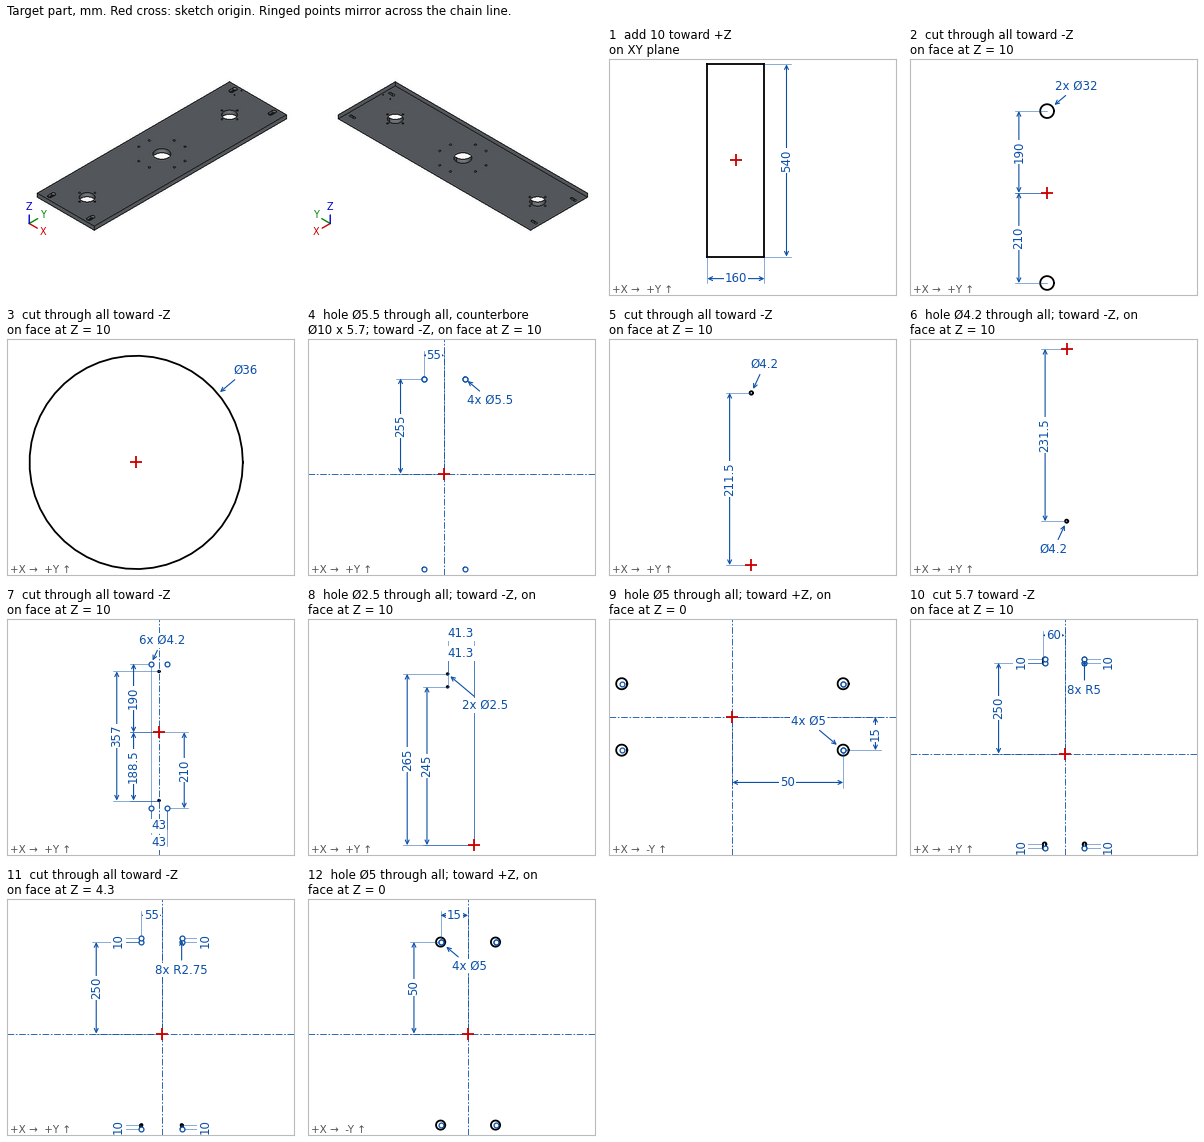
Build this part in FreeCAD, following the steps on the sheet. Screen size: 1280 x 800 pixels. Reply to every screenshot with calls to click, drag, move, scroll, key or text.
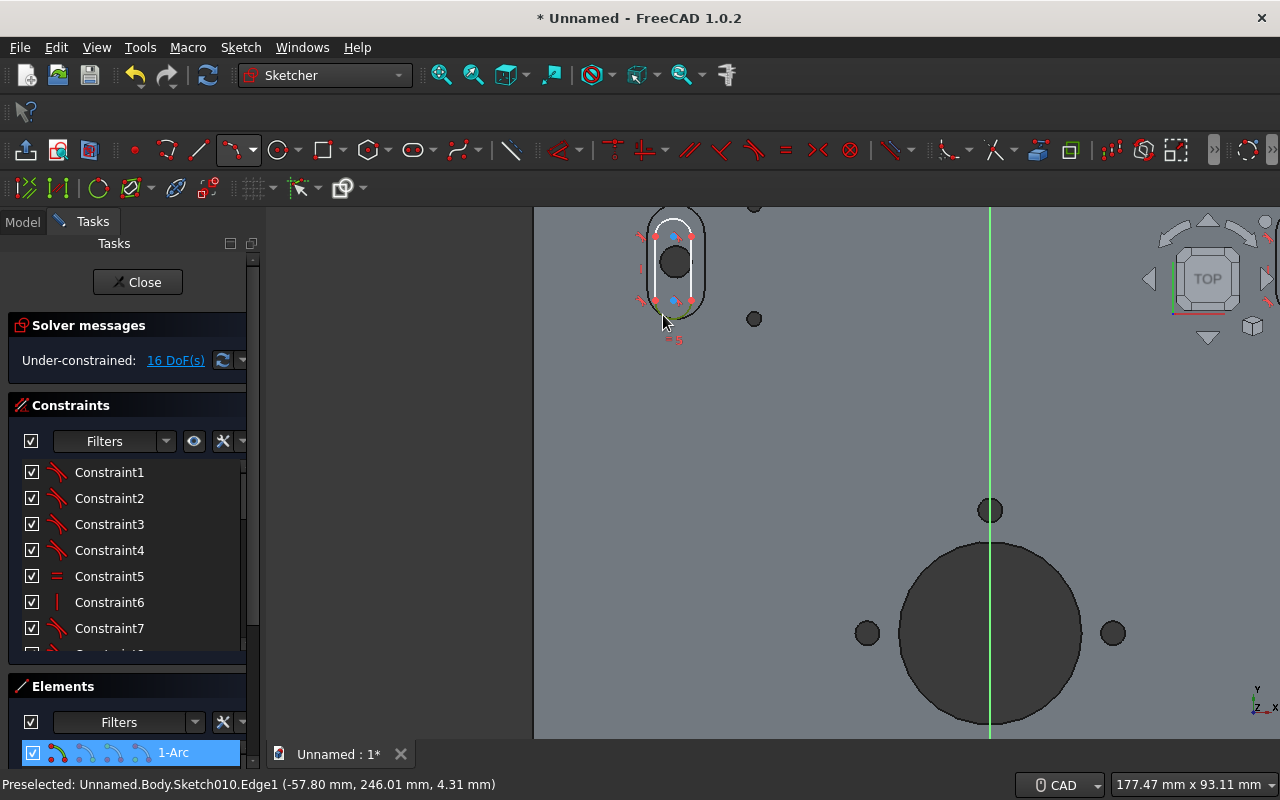
scroll(669, 318, down, 11)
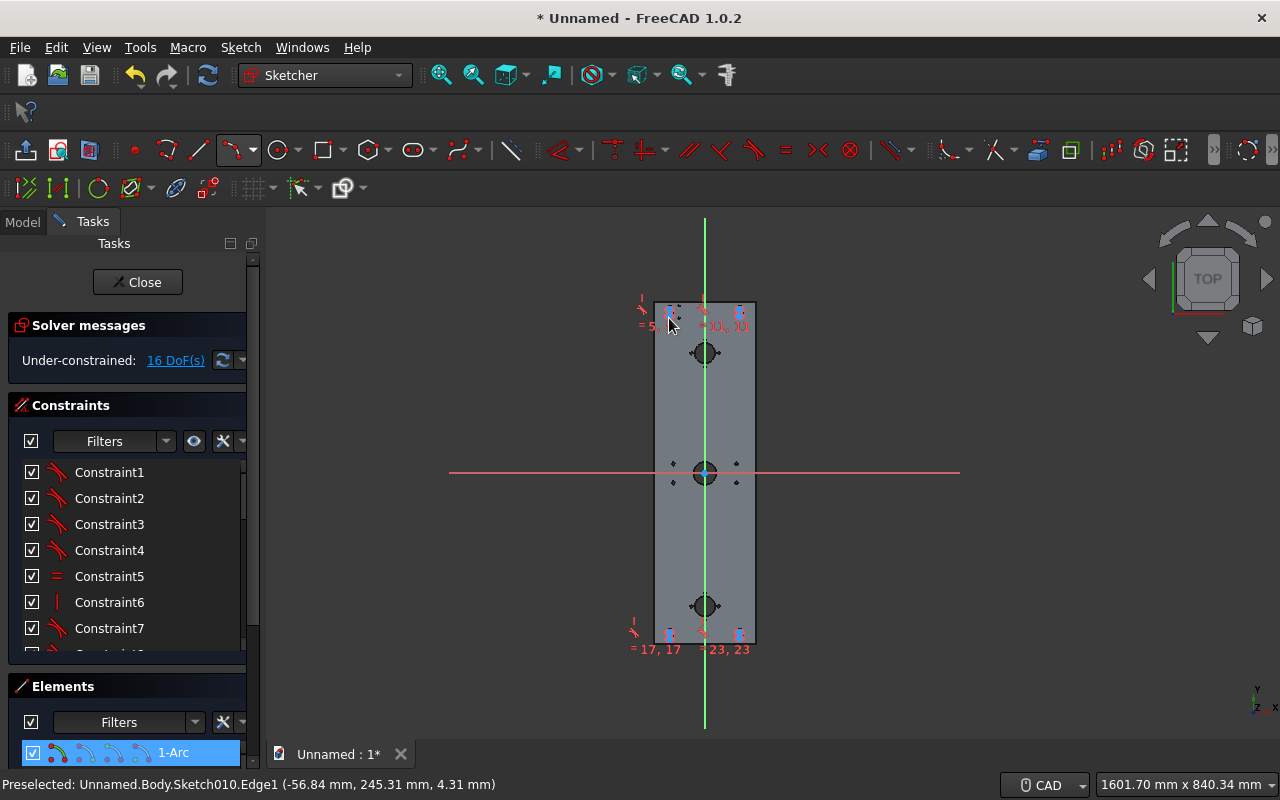
scroll(738, 318, up, 10)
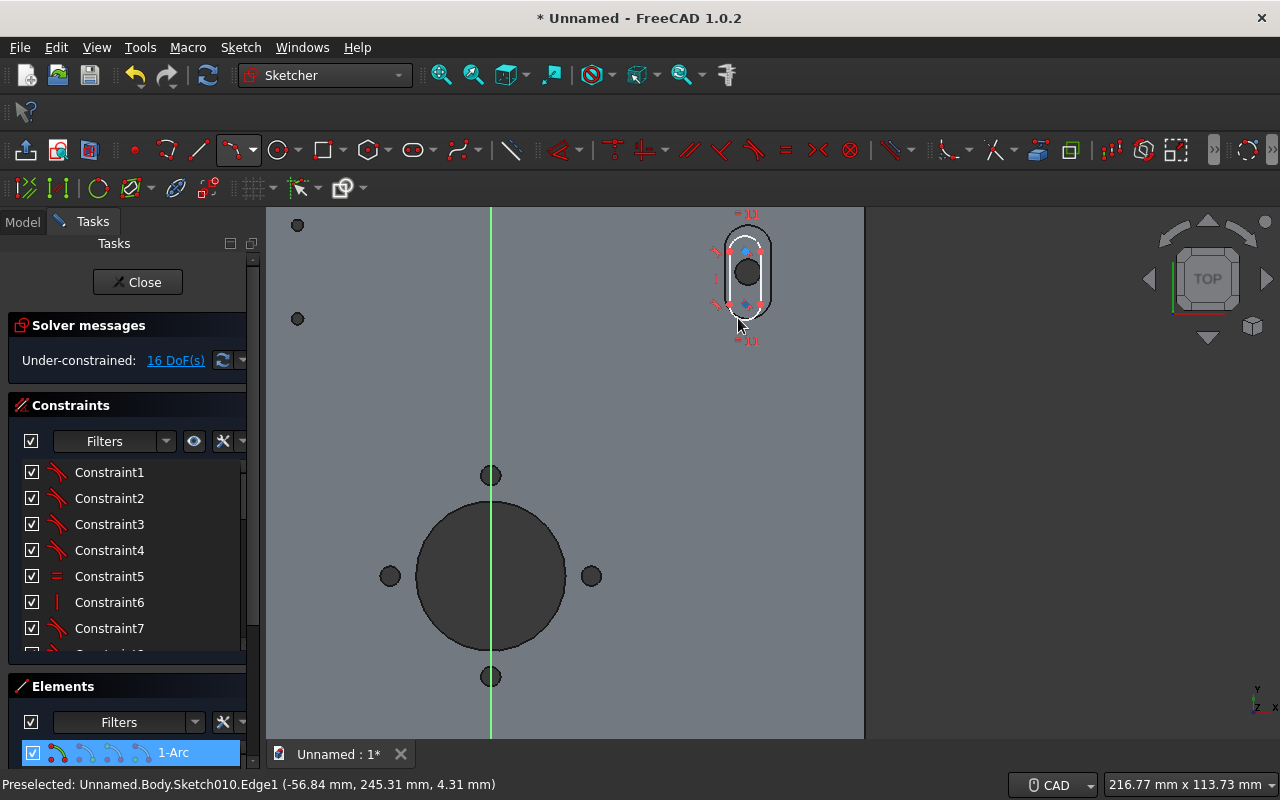
click(736, 317)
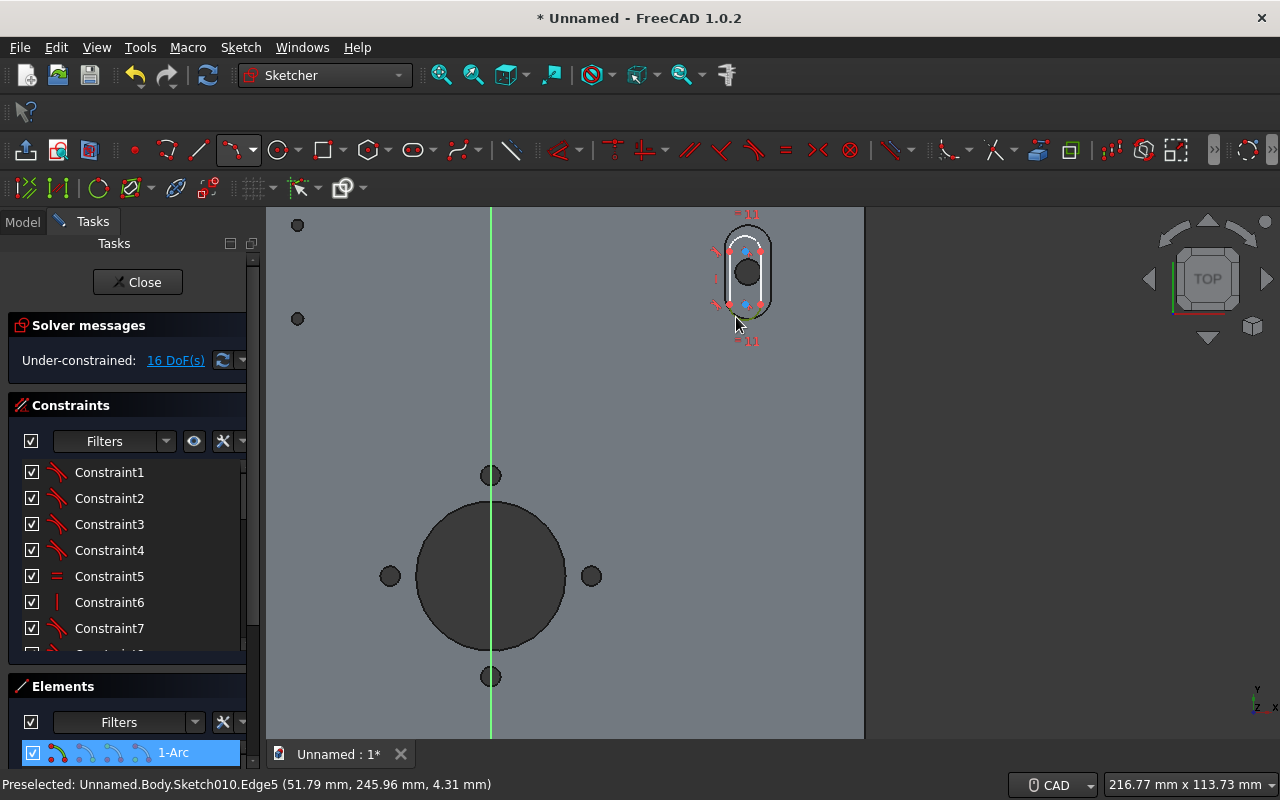
scroll(738, 318, down, 10)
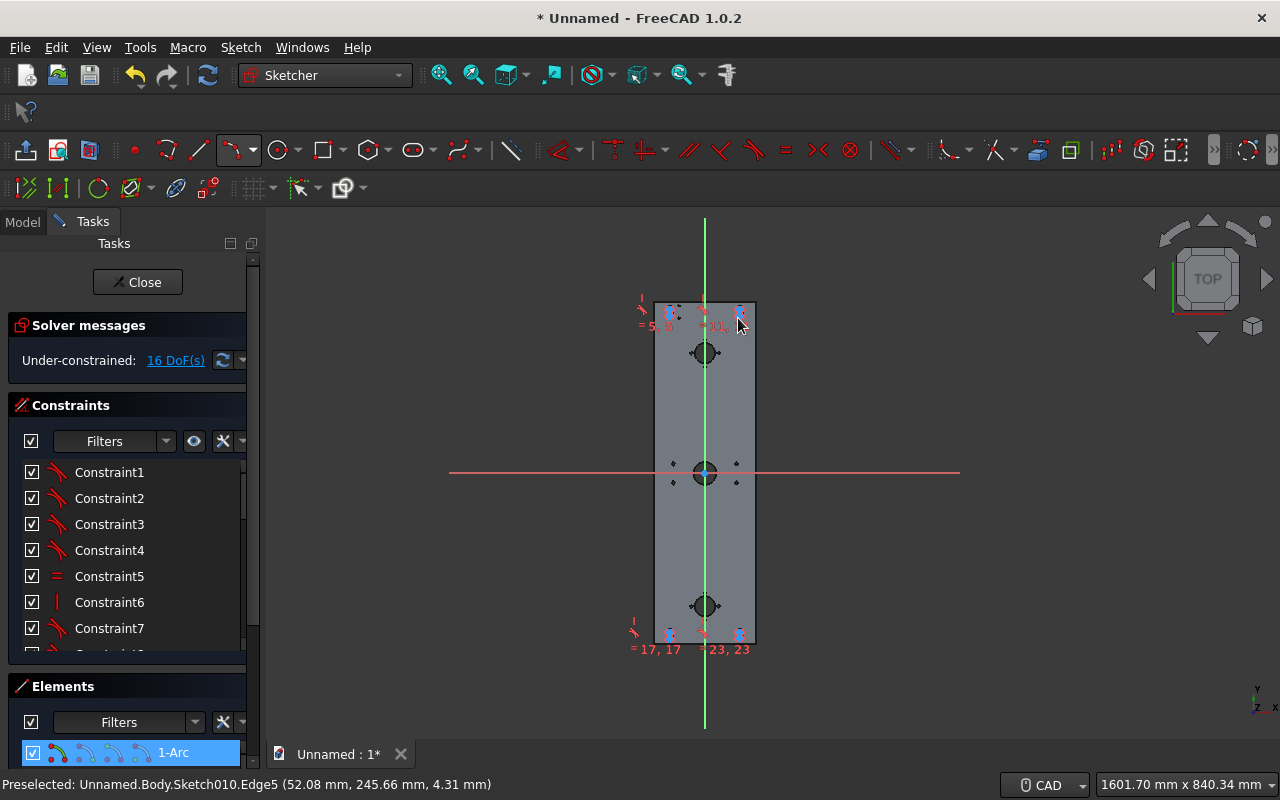
scroll(669, 641, up, 11)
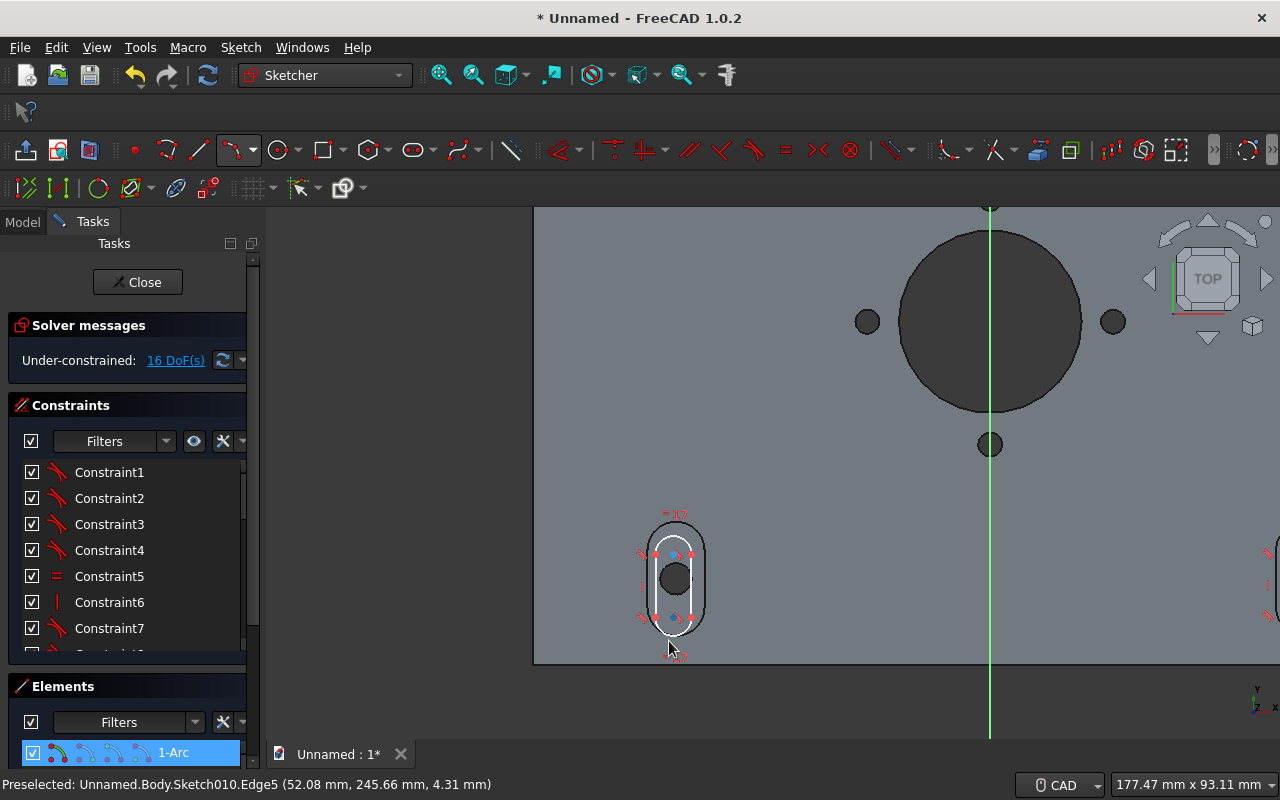
click(663, 633)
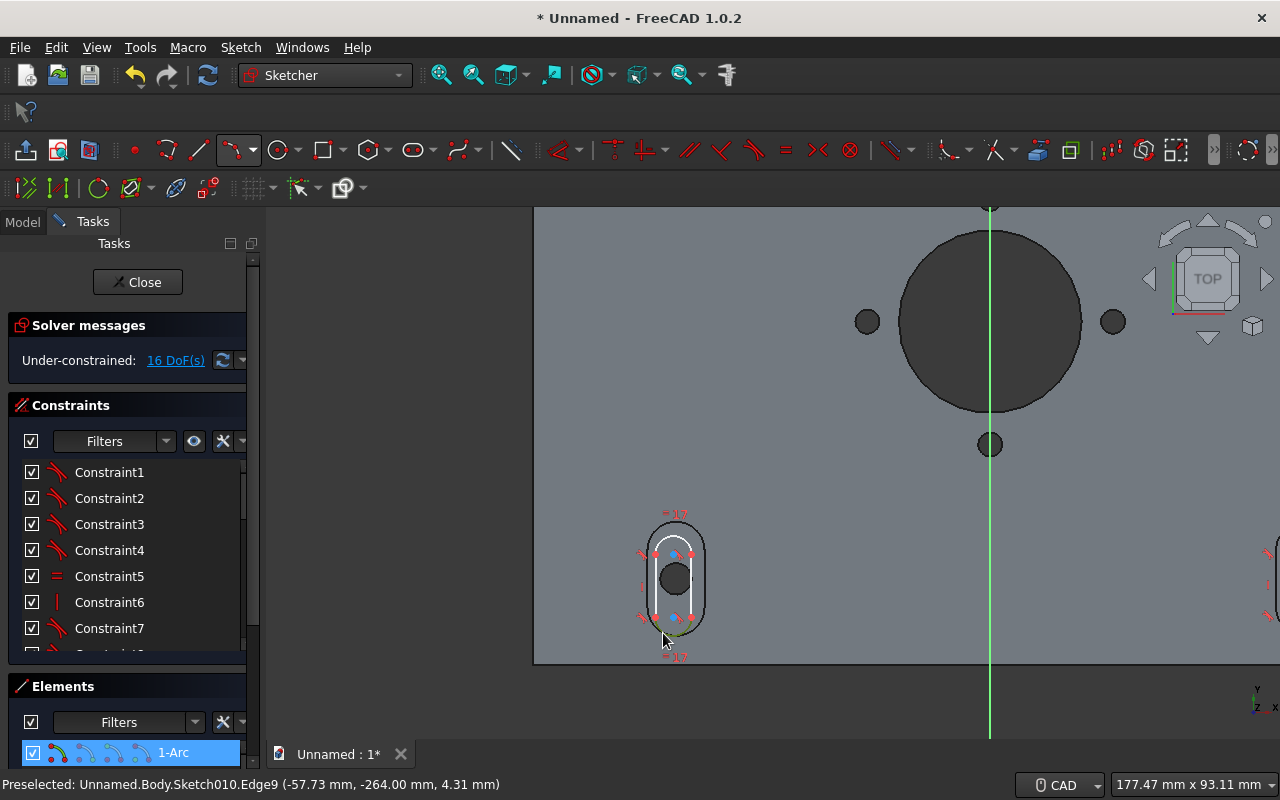
scroll(669, 641, down, 11)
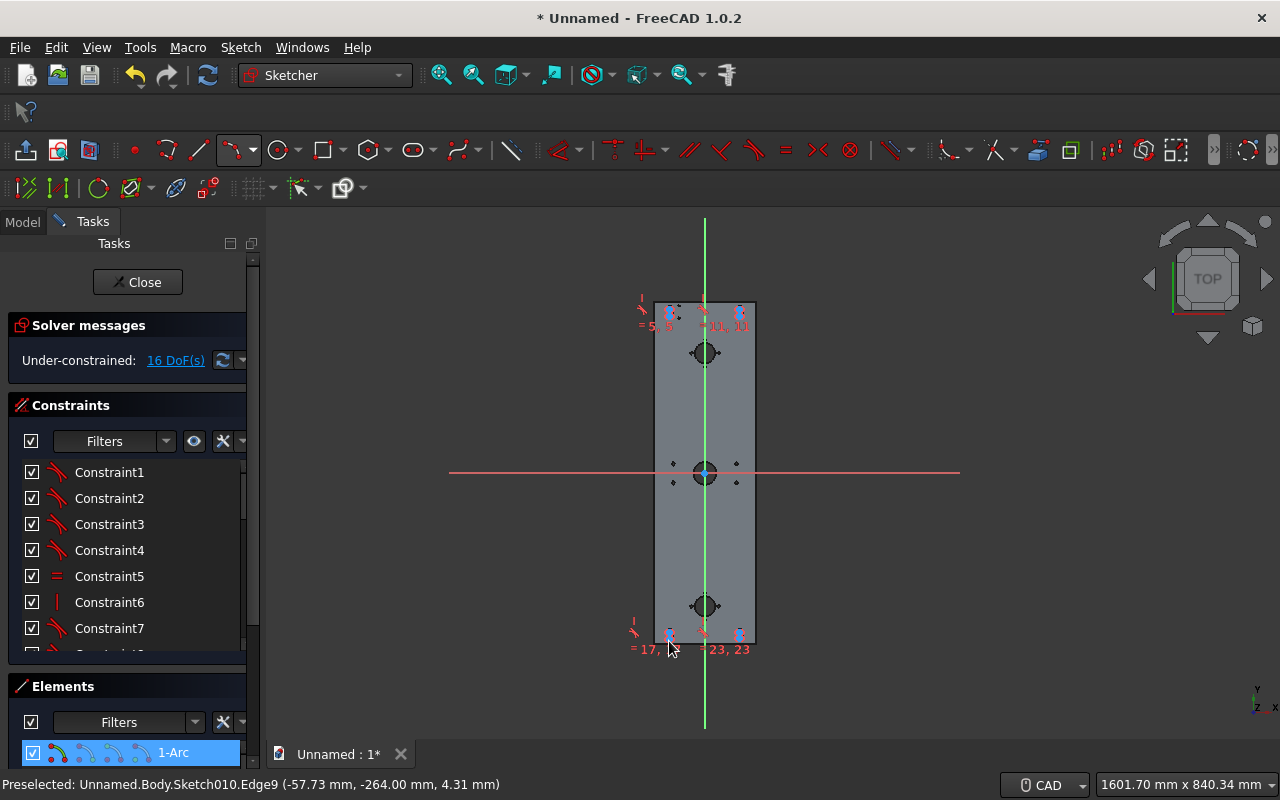
scroll(738, 641, up, 10)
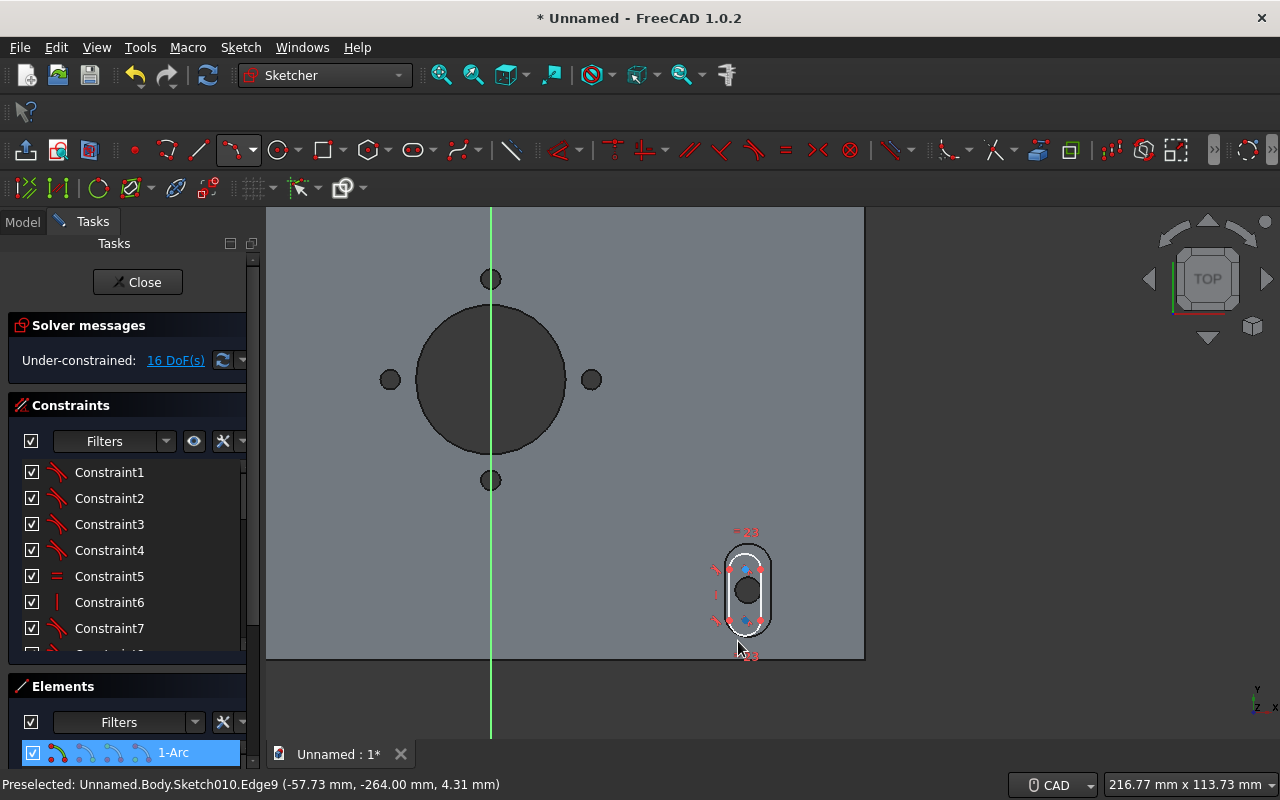
click(736, 633)